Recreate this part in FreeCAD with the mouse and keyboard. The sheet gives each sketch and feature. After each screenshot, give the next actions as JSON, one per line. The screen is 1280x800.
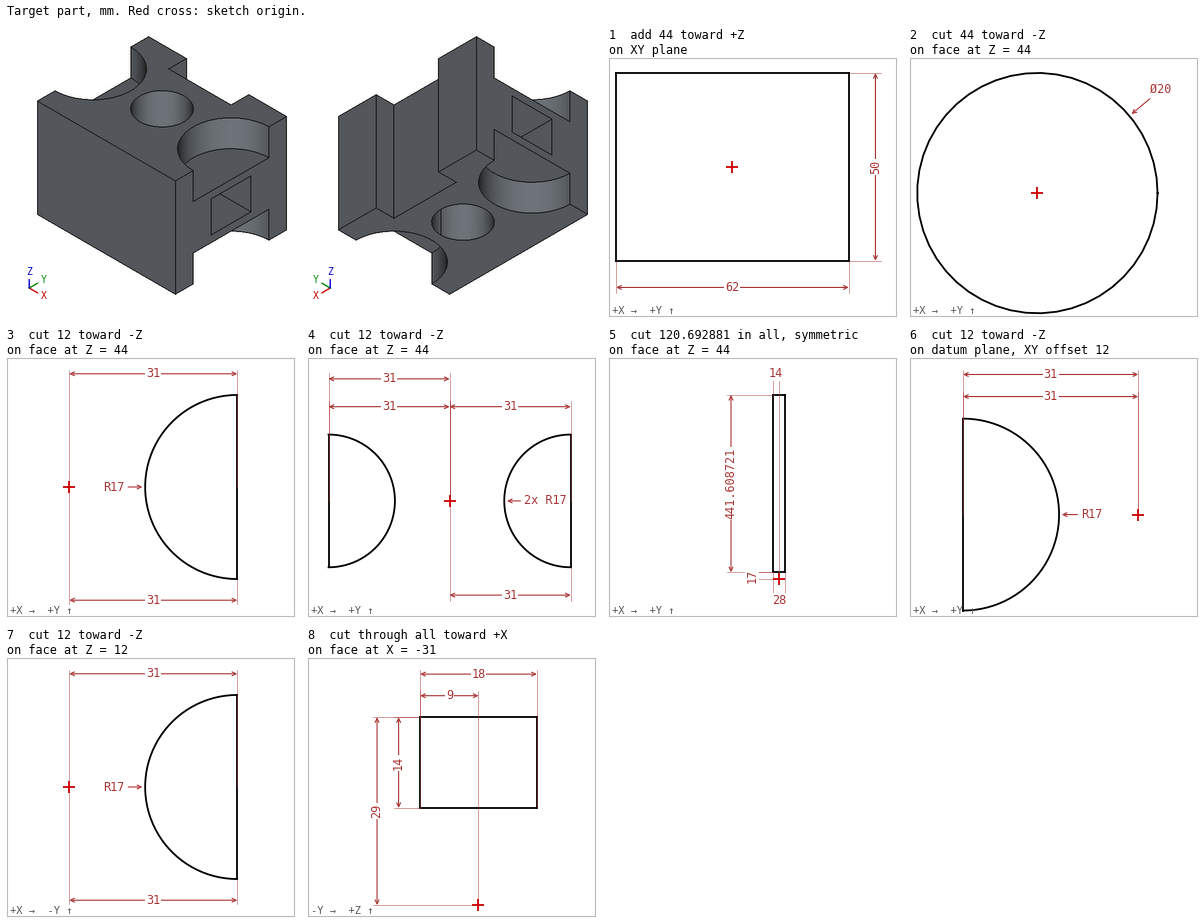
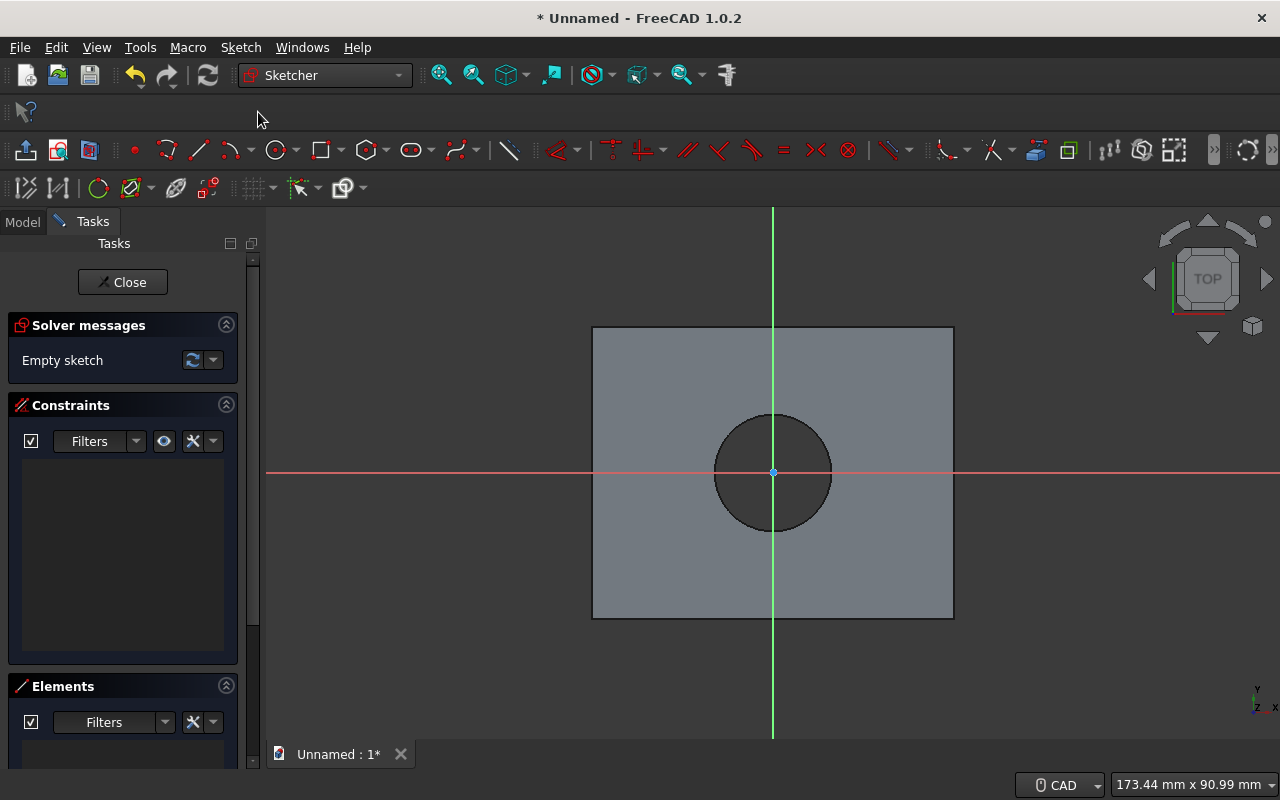
{"action": "scroll", "coordinate": [1057, 473], "scroll_direction": "up", "scroll_amount": 3}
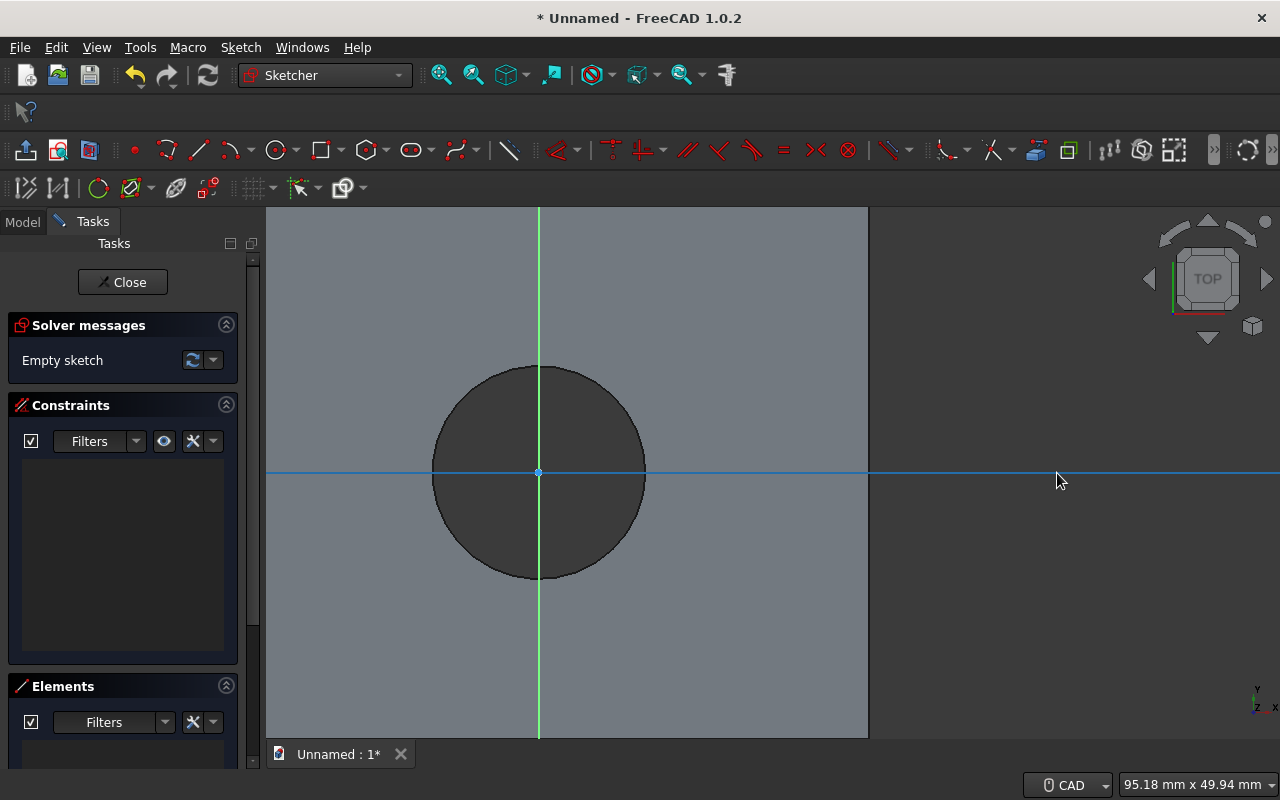
{"action": "key", "text": "g l"}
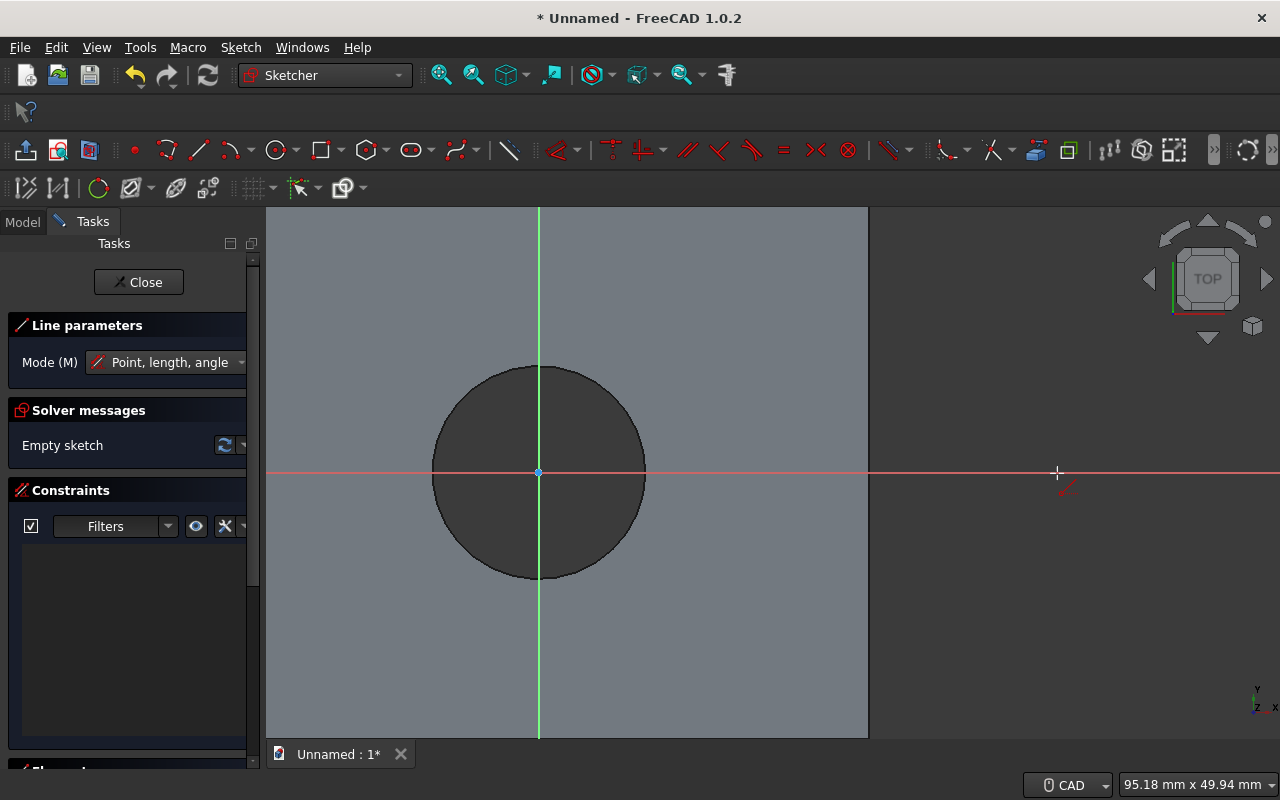
{"action": "left_click", "coordinate": [869, 654]}
{"action": "left_click", "coordinate": [869, 291]}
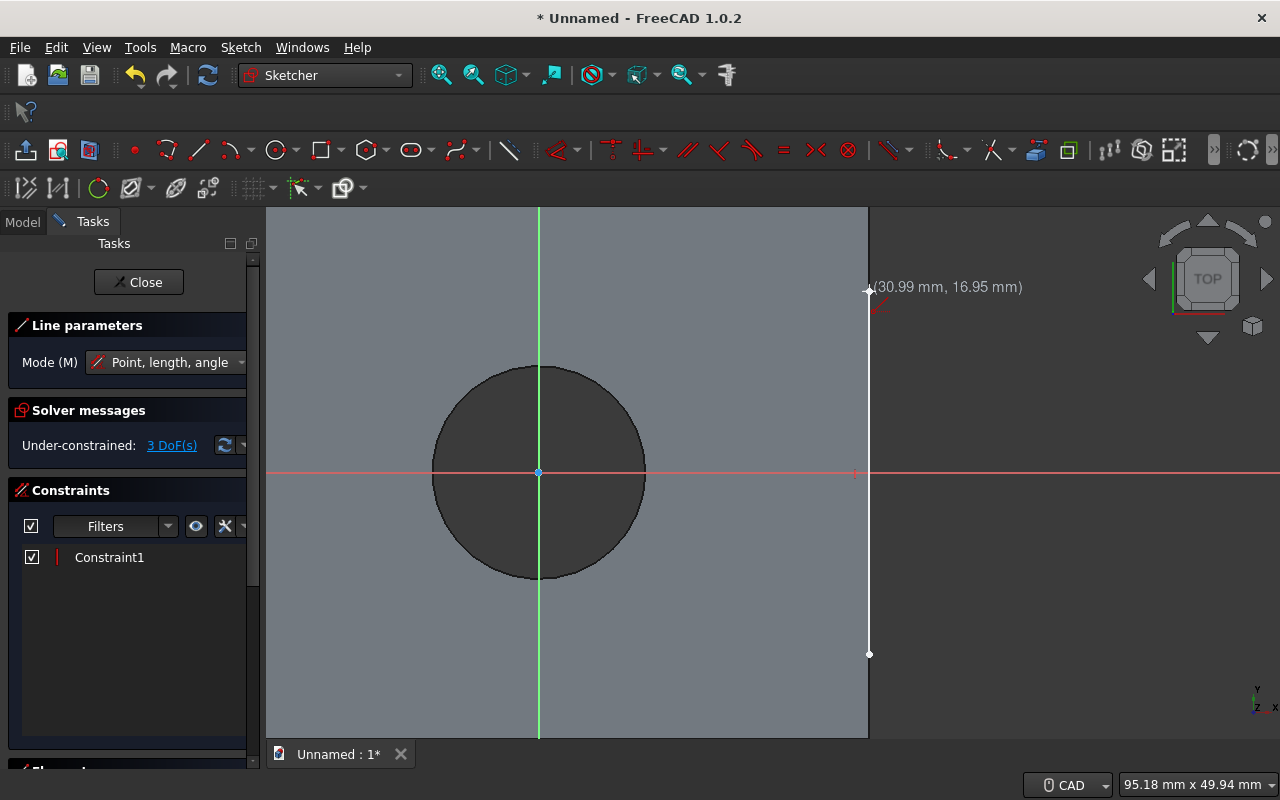
{"action": "key", "text": "g 3 a"}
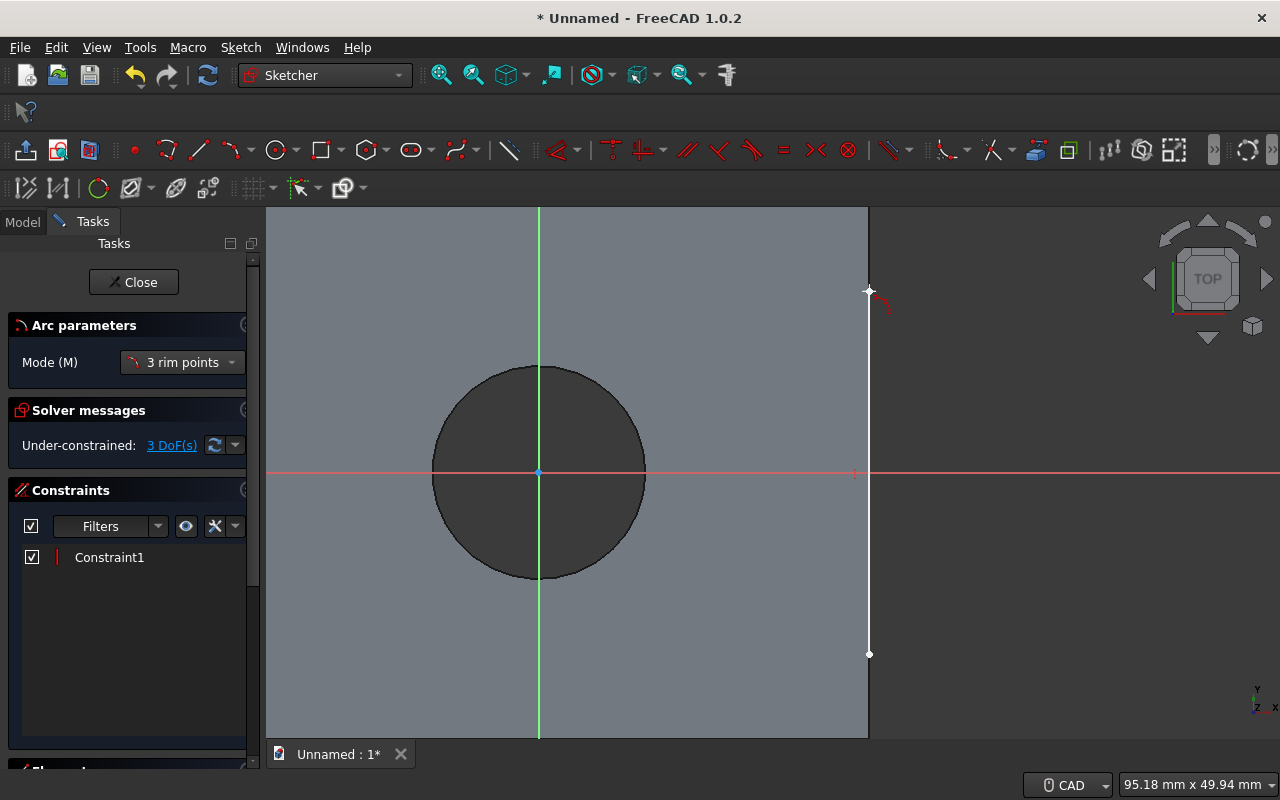
{"action": "left_click", "coordinate": [869, 292]}
{"action": "left_click", "coordinate": [869, 655]}
{"action": "left_click", "coordinate": [697, 417]}
{"action": "key", "text": "Escape"}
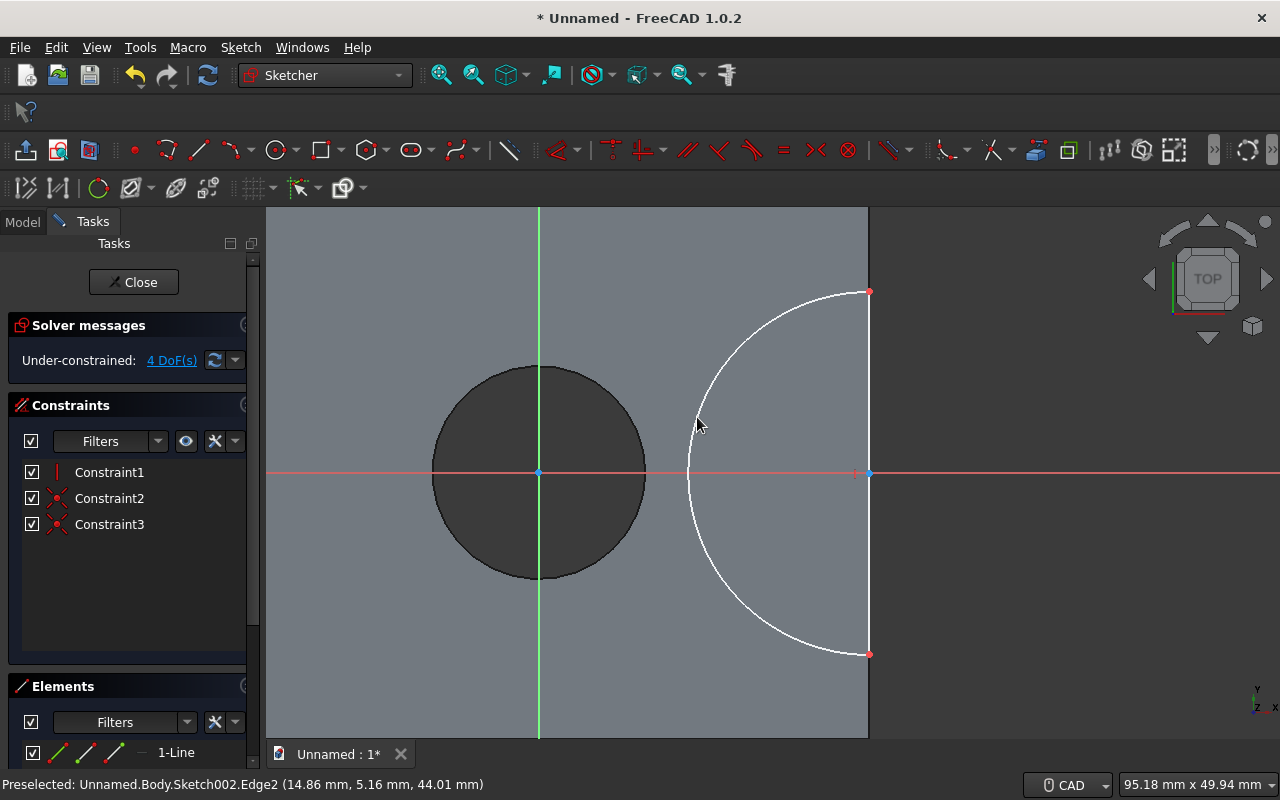
{"action": "left_click", "coordinate": [870, 473]}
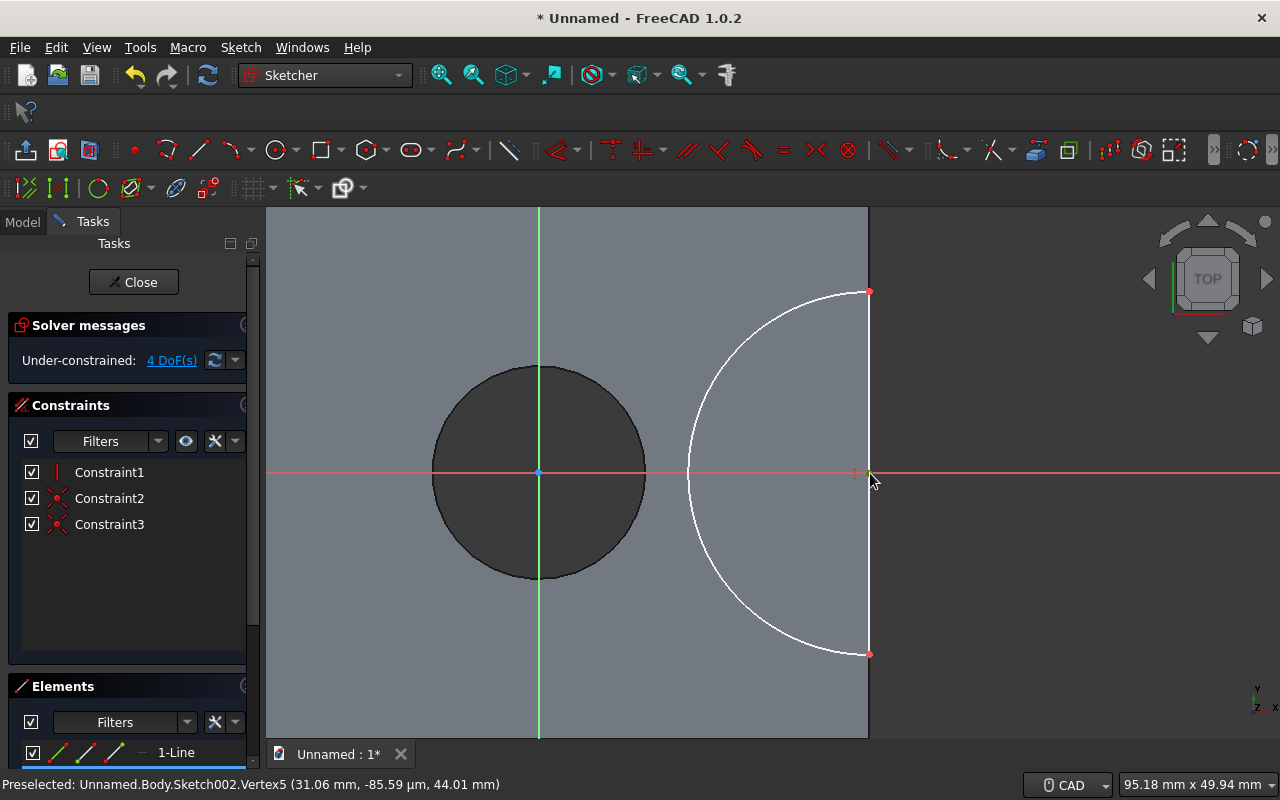
{"action": "left_click", "coordinate": [353, 473]}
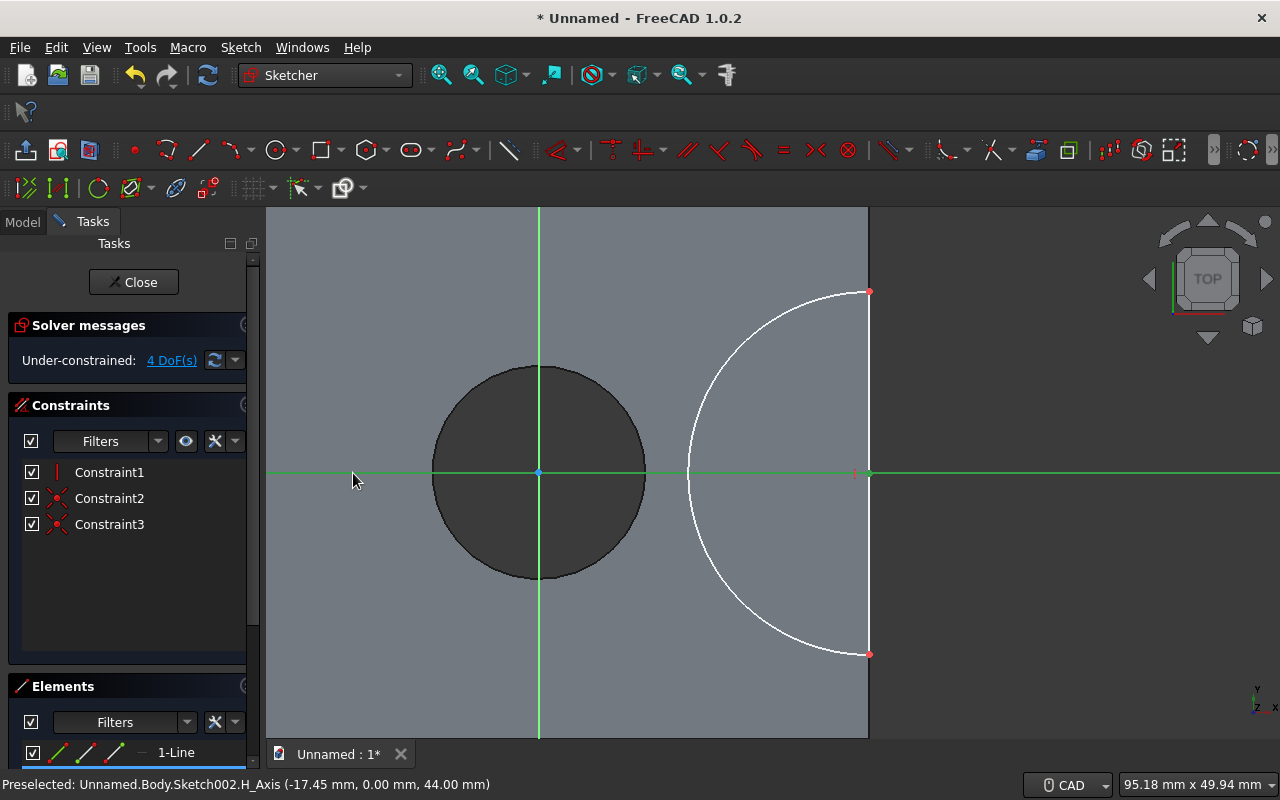
{"action": "key", "text": "c"}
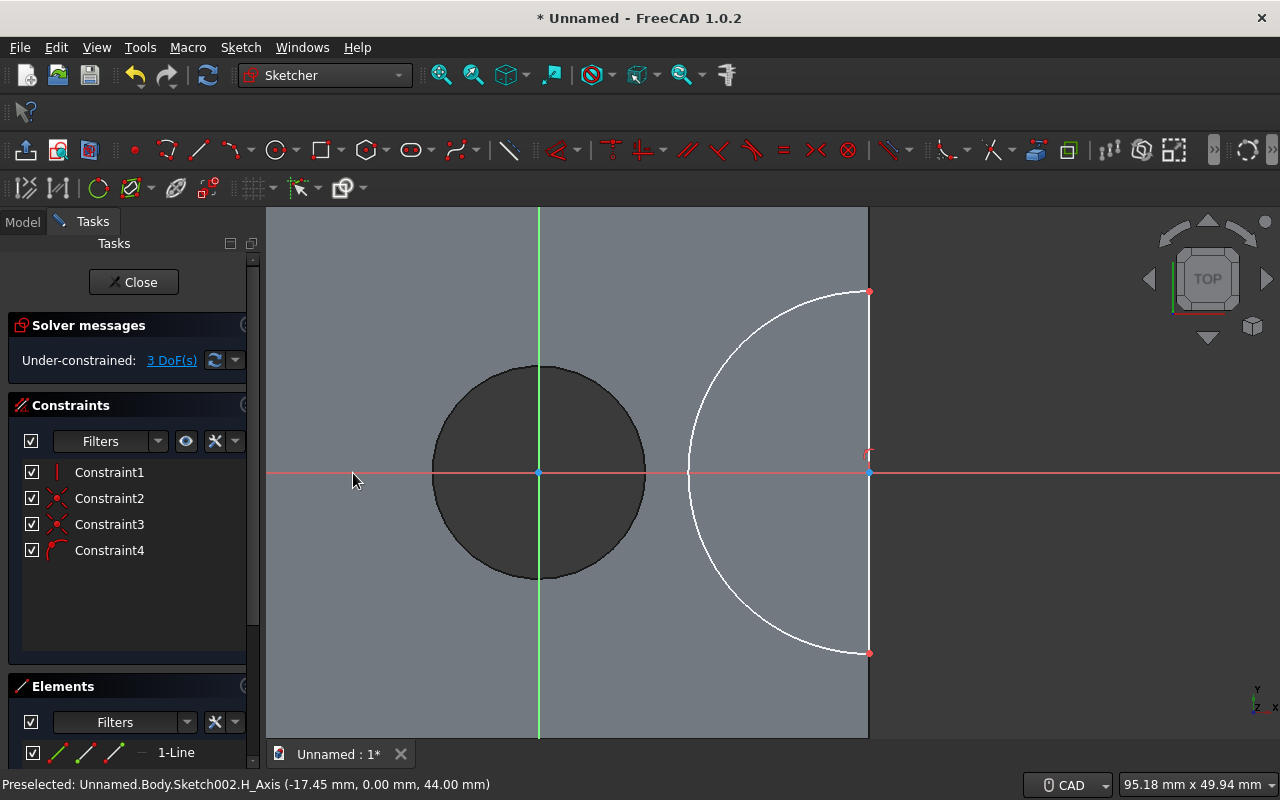
{"action": "key", "text": "d"}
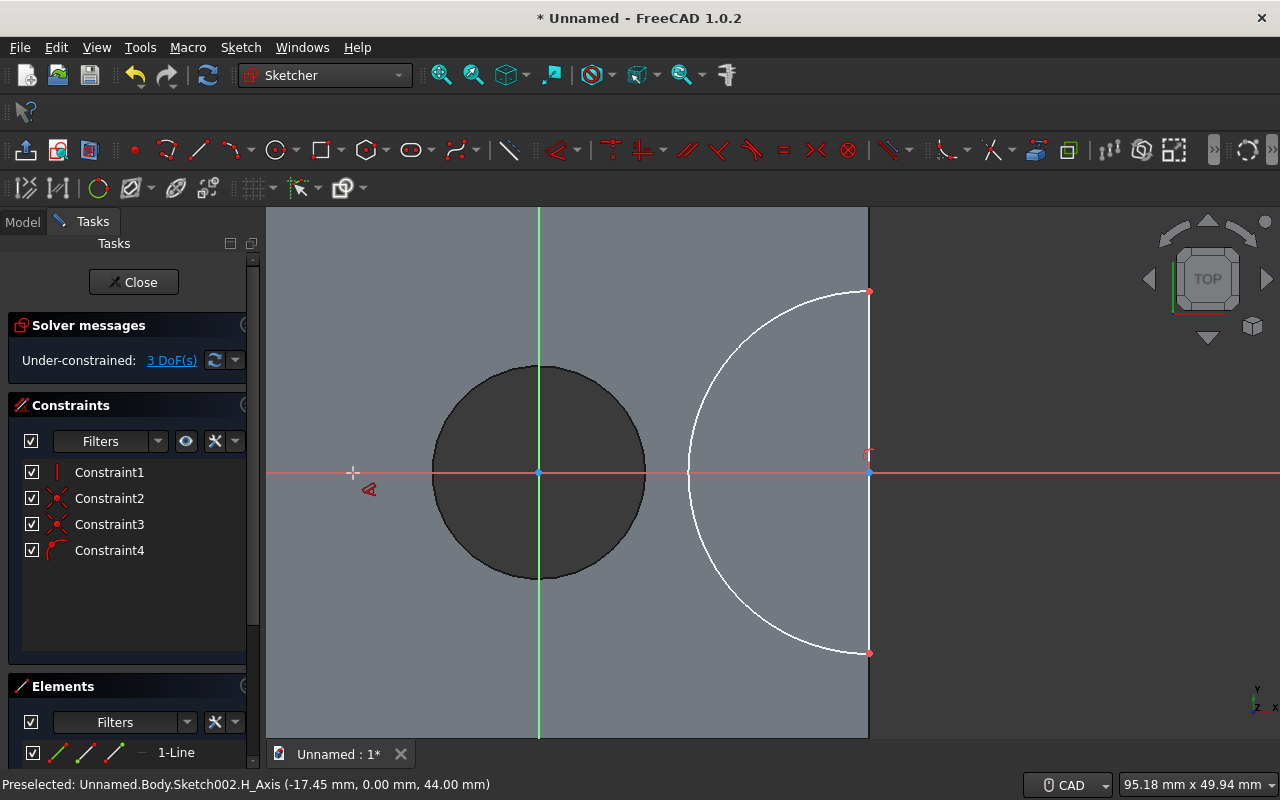
{"action": "left_click", "coordinate": [723, 366]}
{"action": "left_click", "coordinate": [697, 347]}